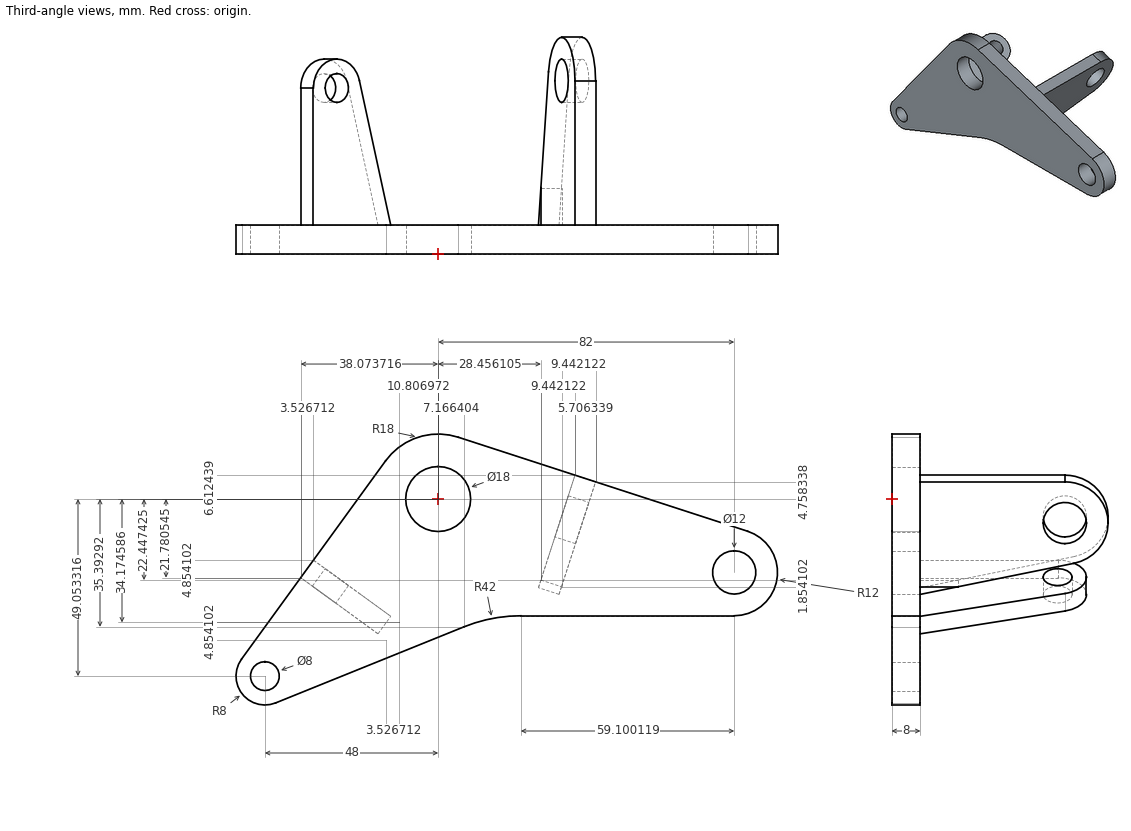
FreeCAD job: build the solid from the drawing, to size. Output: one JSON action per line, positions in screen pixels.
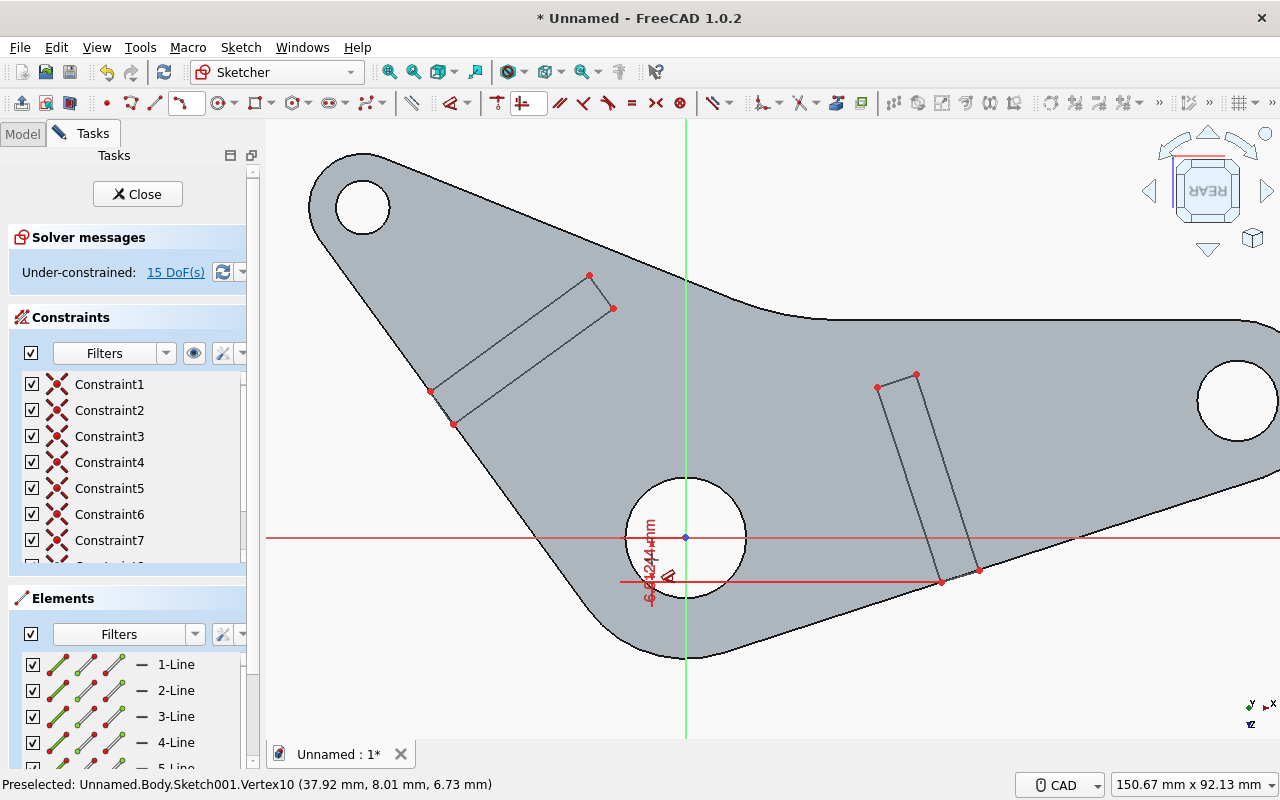
{"action": "scroll", "coordinate": [979, 571], "scroll_direction": "up", "scroll_amount": 2}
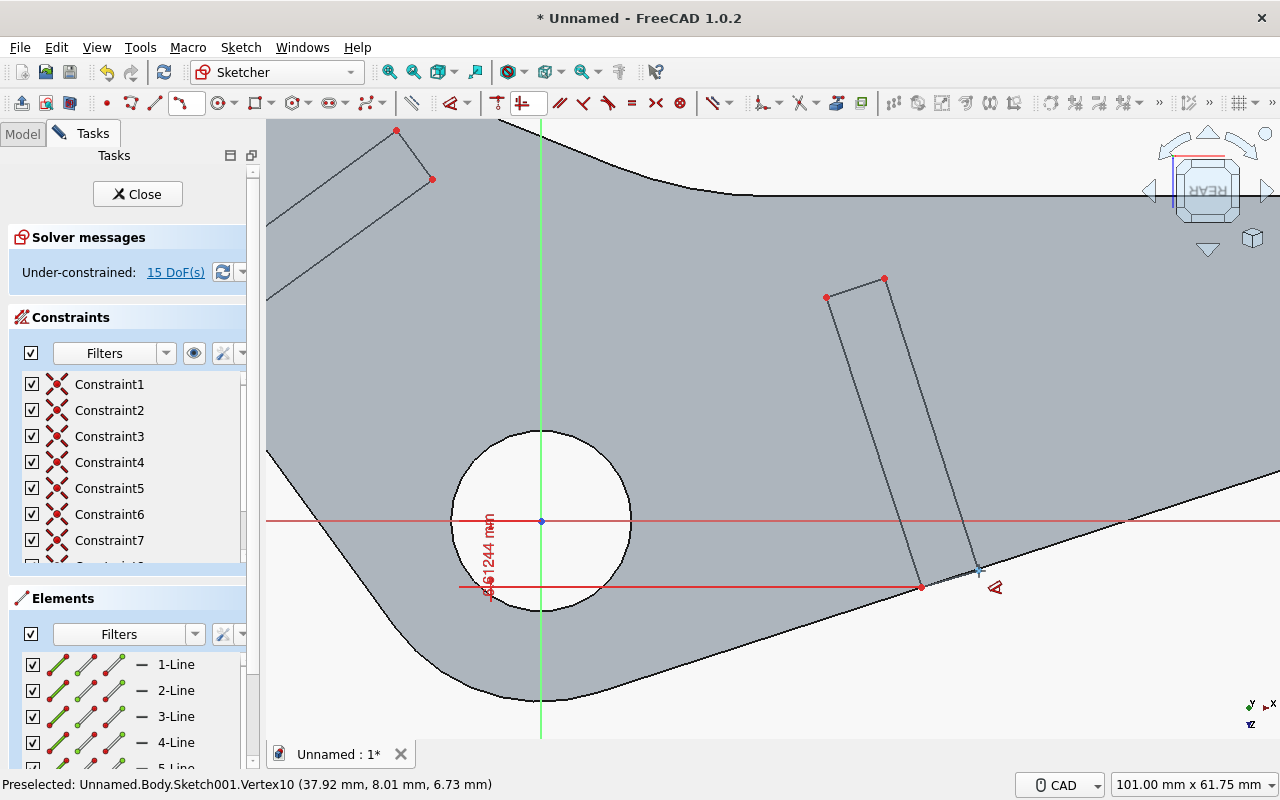
{"action": "left_click", "coordinate": [979, 571]}
{"action": "left_click", "coordinate": [1013, 546]}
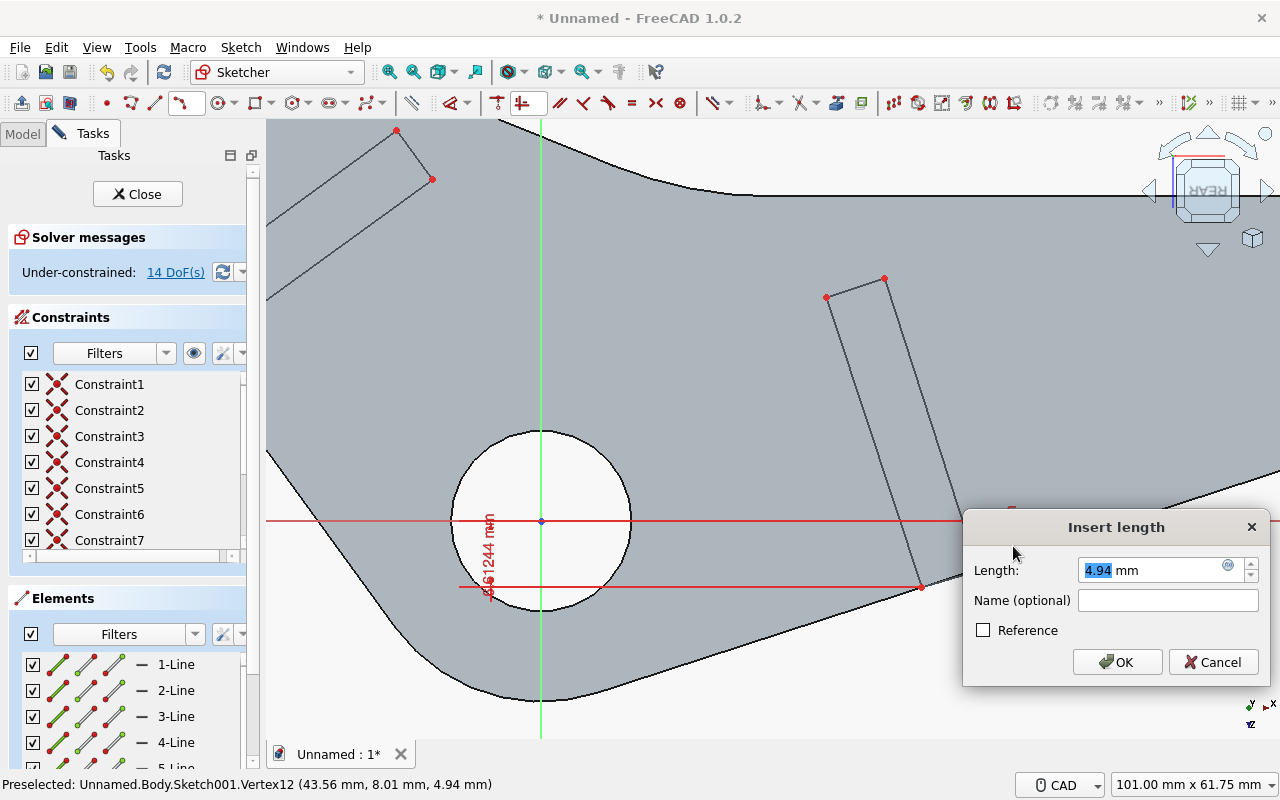
{"action": "type", "text": "4.758338"}
{"action": "key", "text": "Return"}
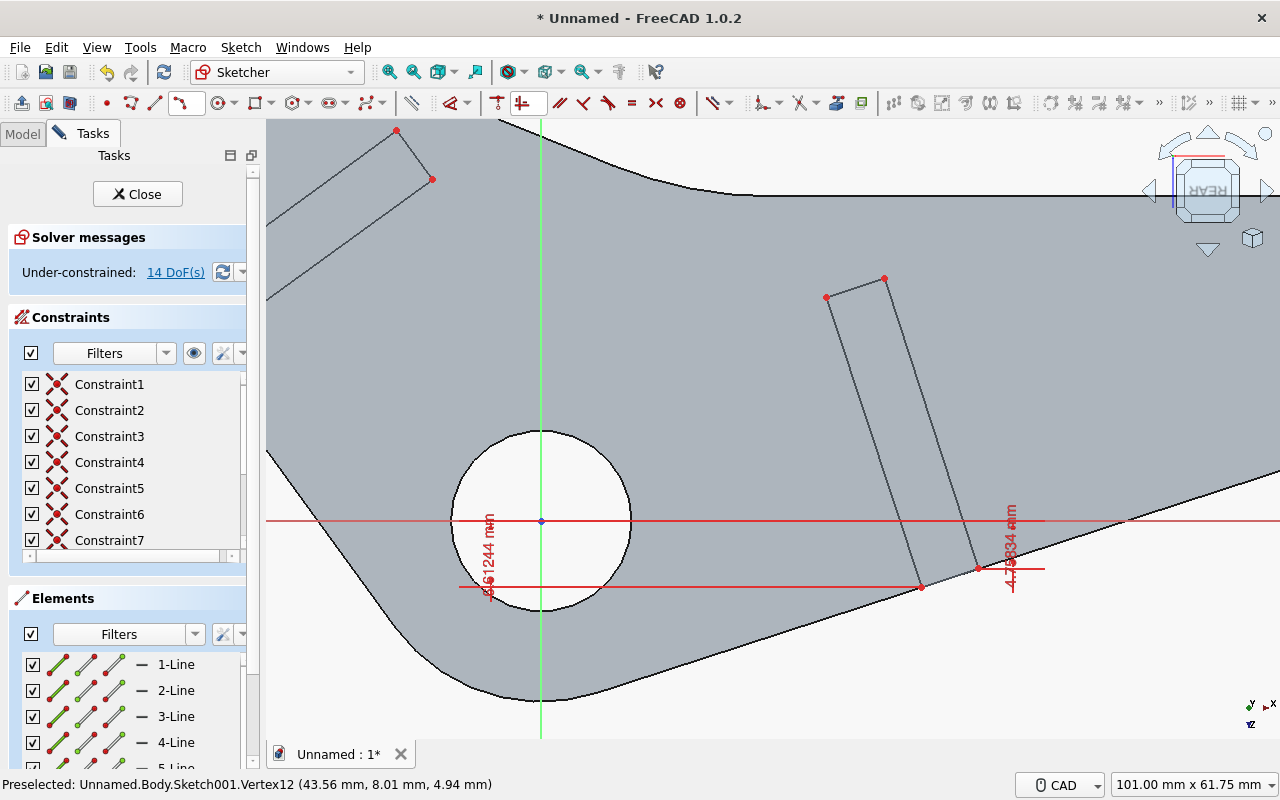
{"action": "left_click", "coordinate": [422, 165]}
{"action": "left_click", "coordinate": [415, 214]}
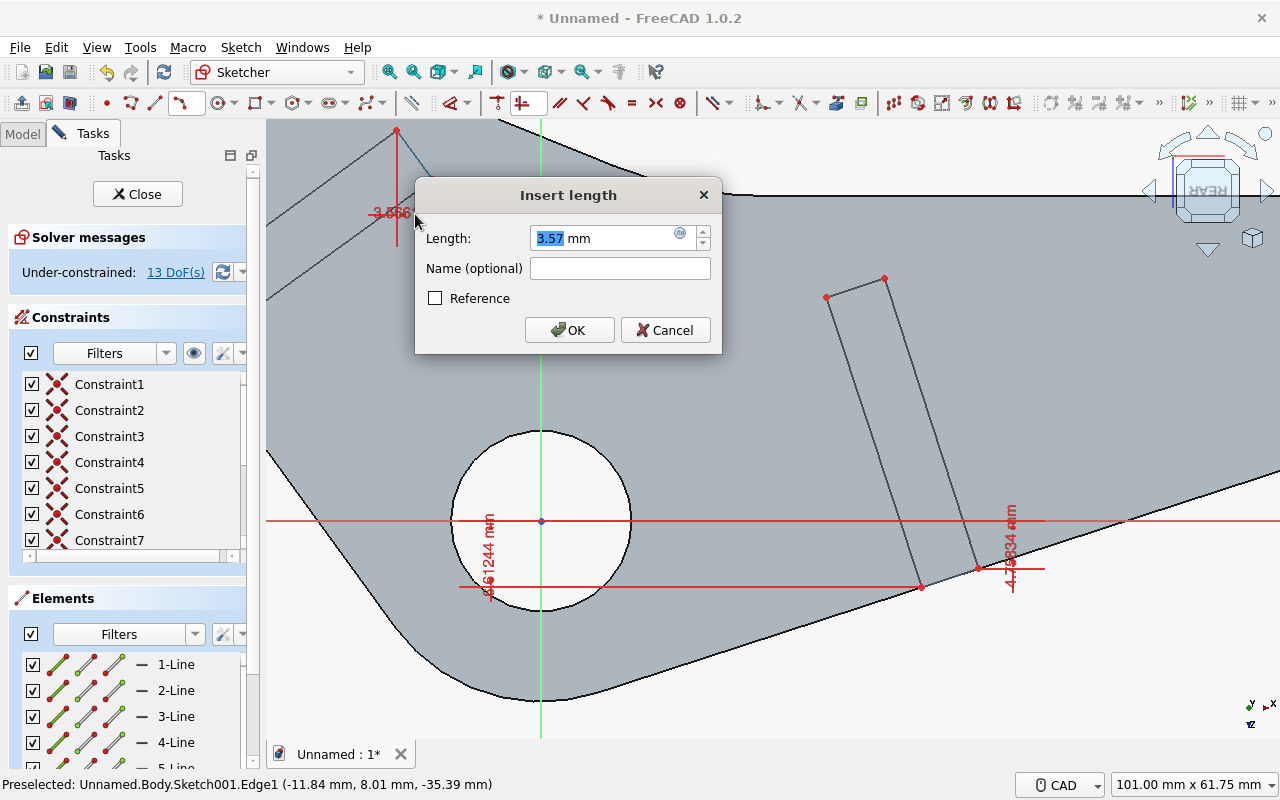
{"action": "type", "text": "3.526712"}
{"action": "key", "text": "Return"}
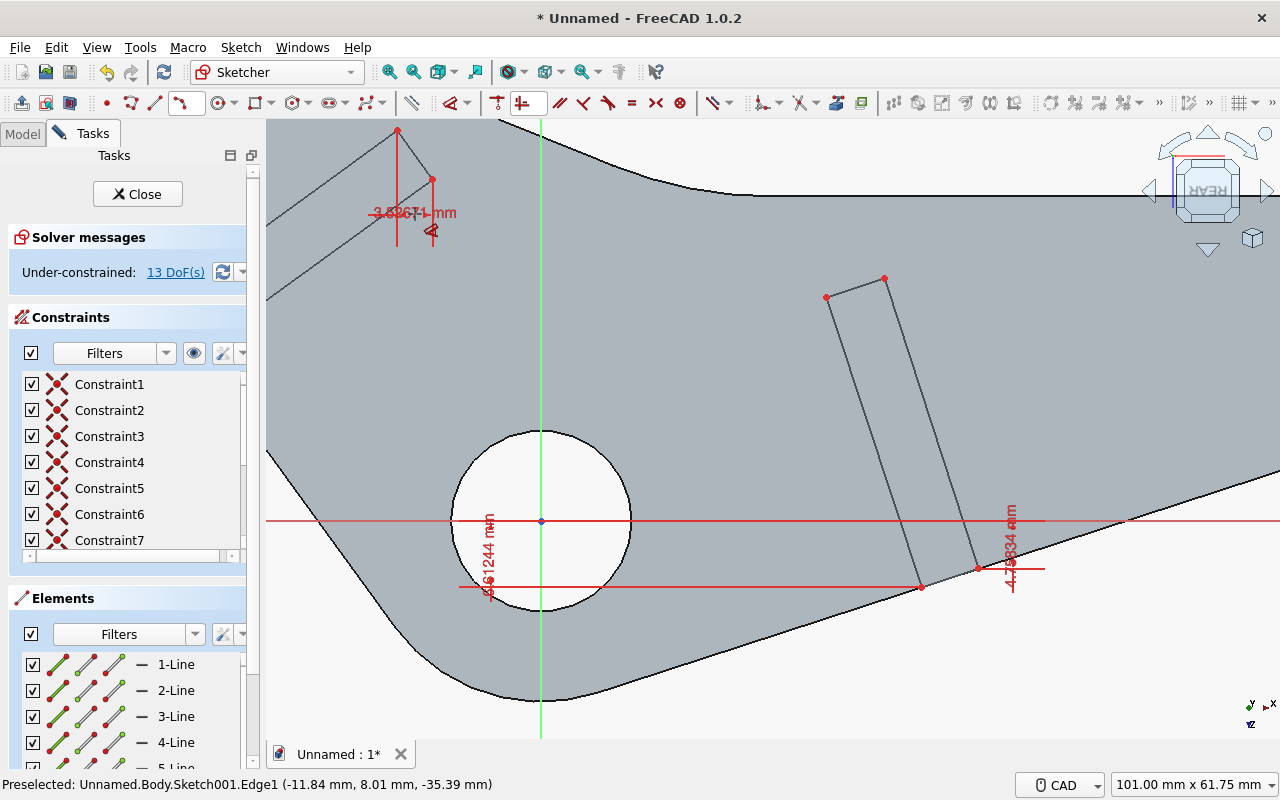
{"action": "left_click", "coordinate": [422, 165]}
{"action": "left_click", "coordinate": [363, 175]}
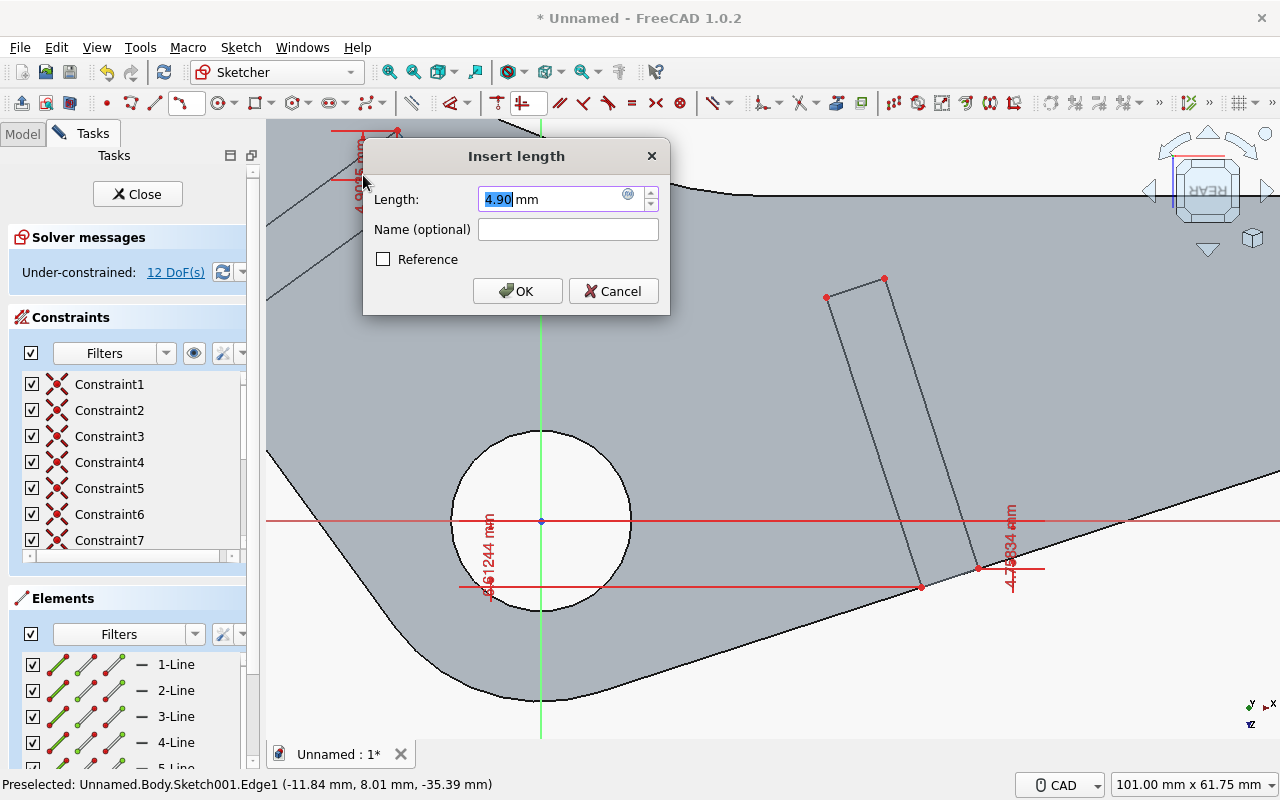
{"action": "type", "text": "4.854102"}
{"action": "key", "text": "Return"}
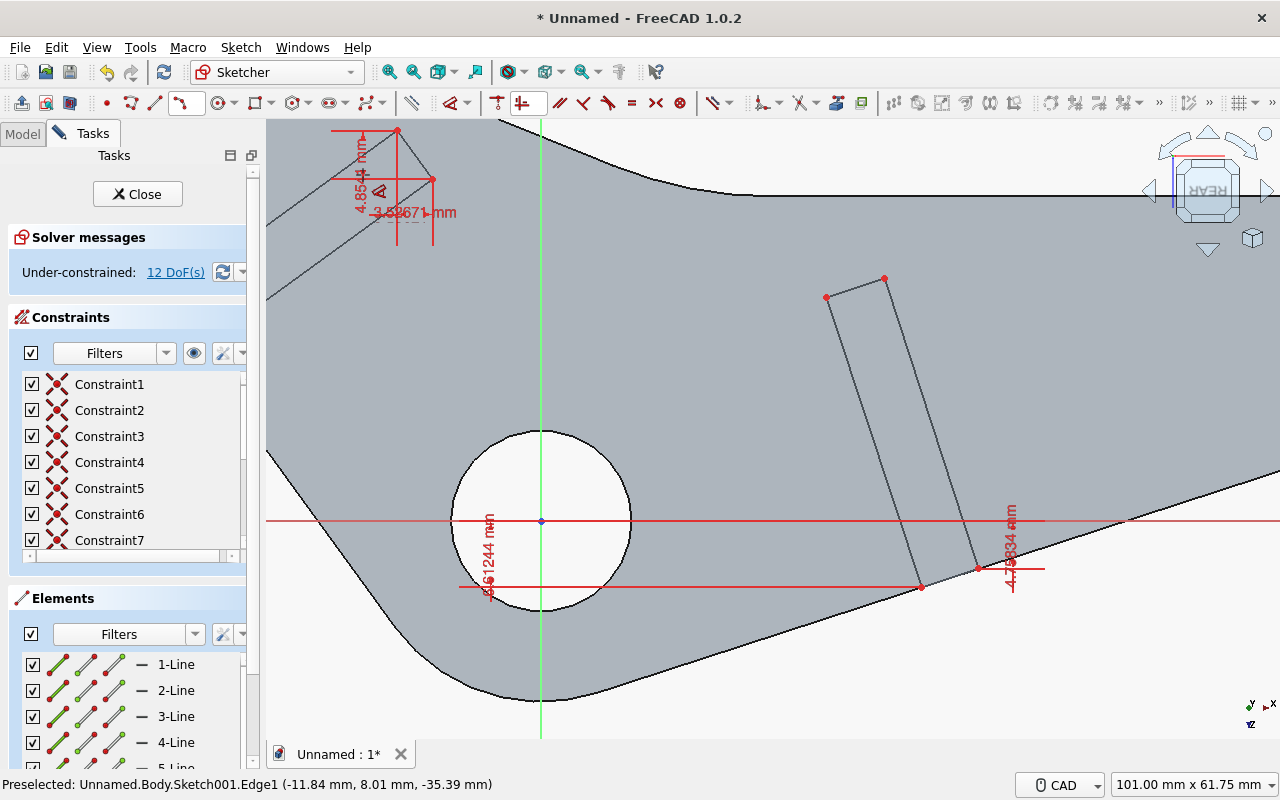
{"action": "scroll", "coordinate": [980, 573], "scroll_direction": "down", "scroll_amount": 2}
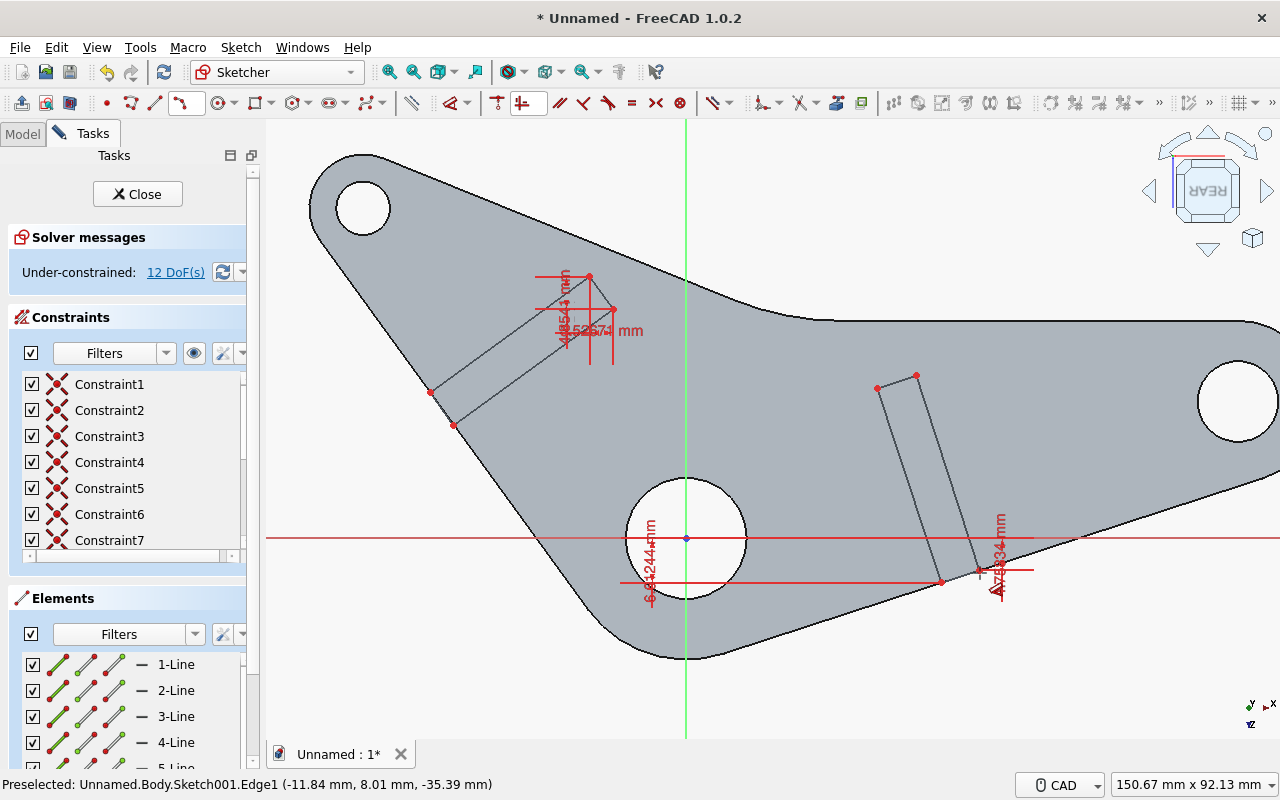
{"action": "scroll", "coordinate": [437, 403], "scroll_direction": "up", "scroll_amount": 3}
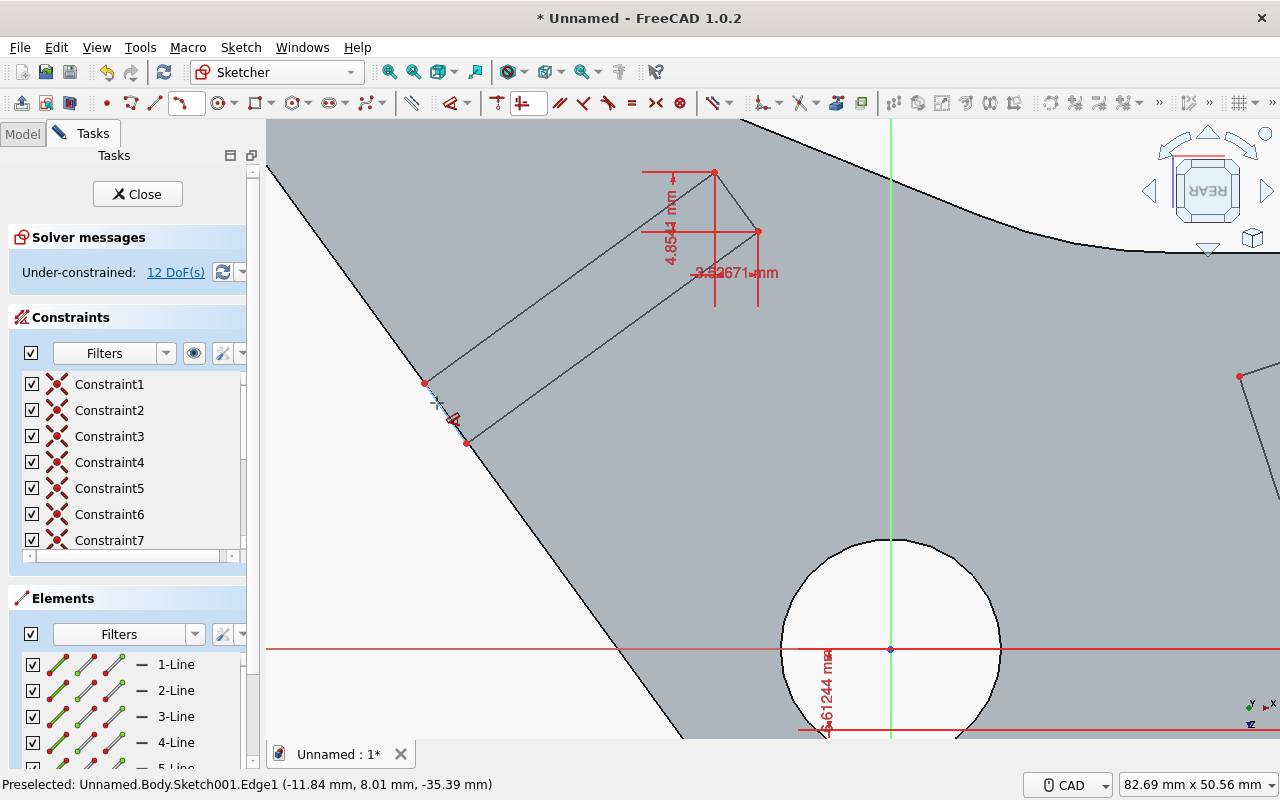
{"action": "left_click", "coordinate": [437, 402]}
{"action": "left_click", "coordinate": [446, 350]}